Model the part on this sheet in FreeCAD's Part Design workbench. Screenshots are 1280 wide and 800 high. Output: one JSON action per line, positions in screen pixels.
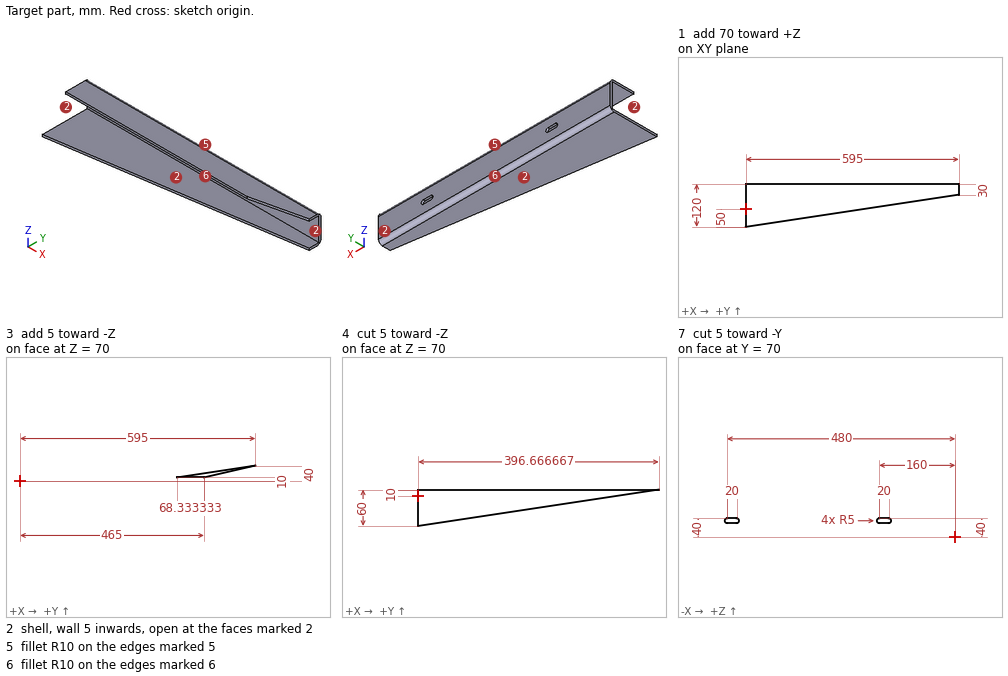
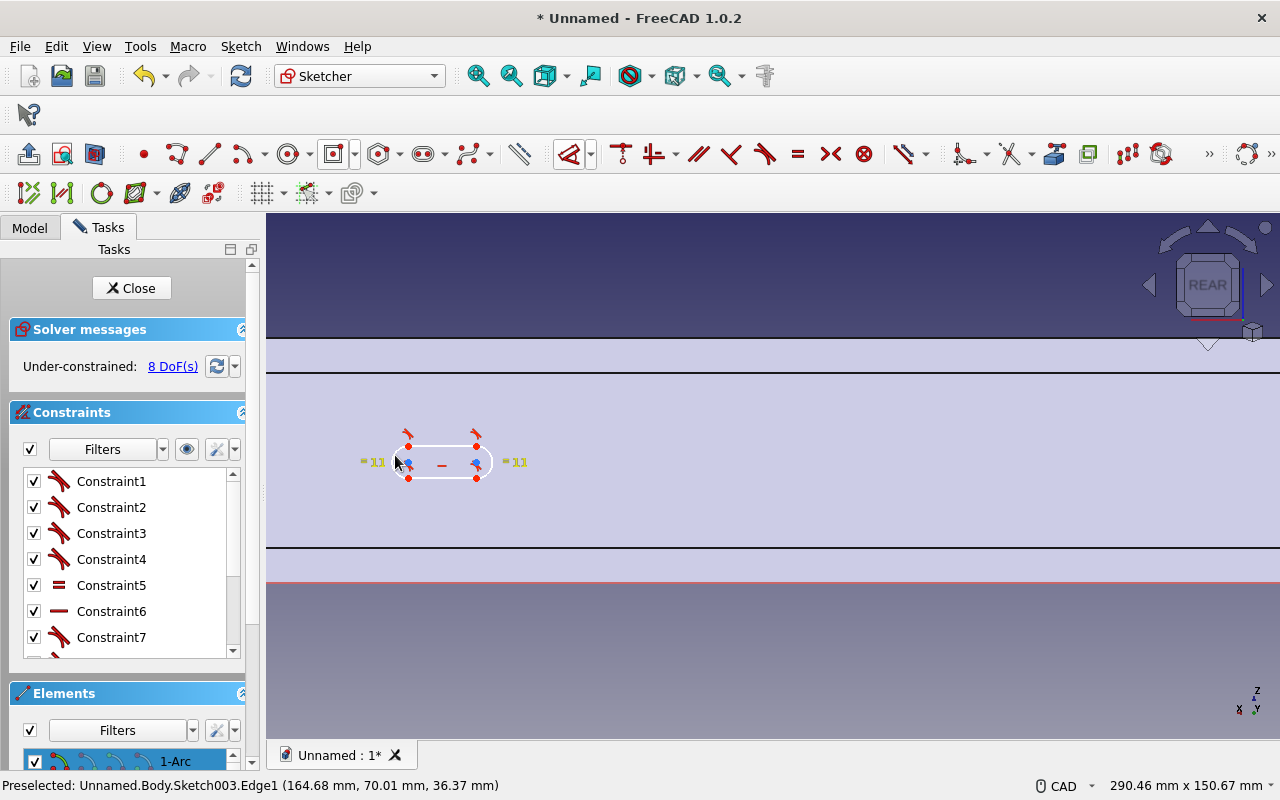
{"action": "left_click", "coordinate": [395, 453]}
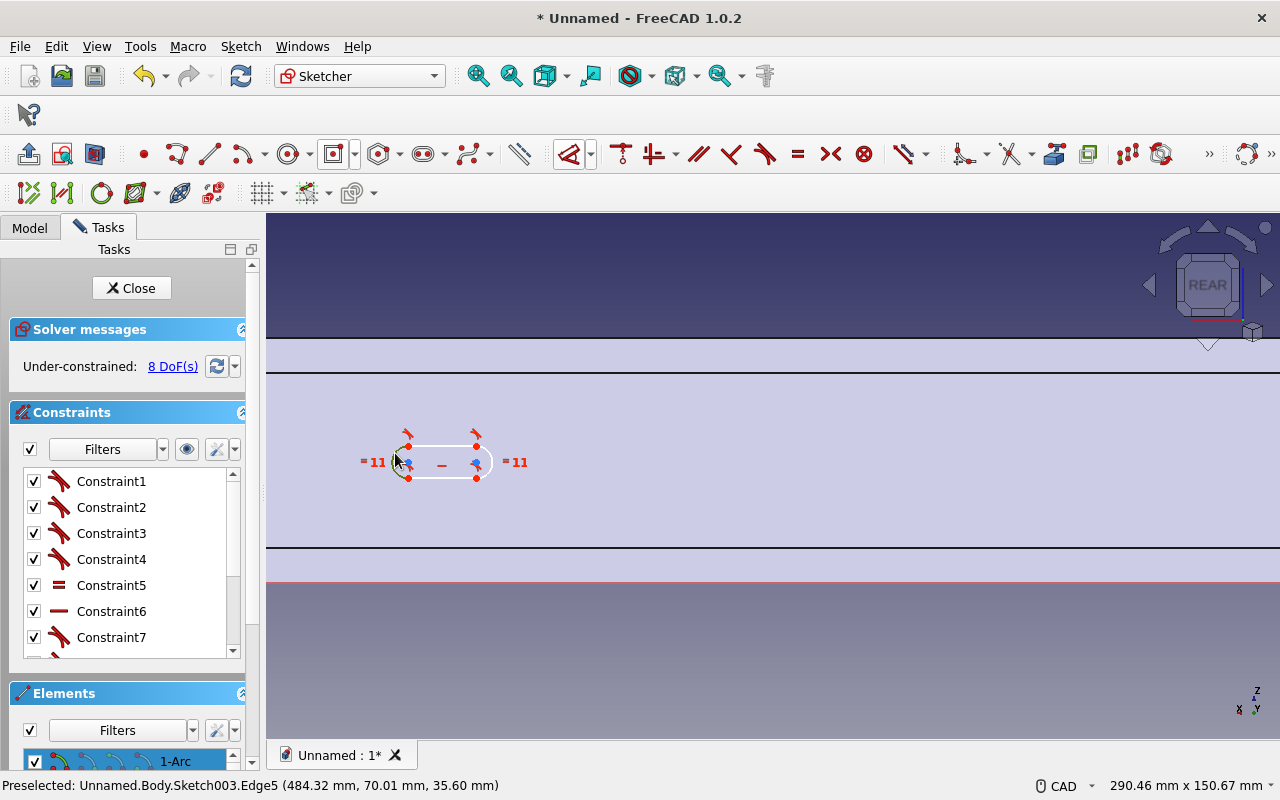
{"action": "left_click", "coordinate": [798, 154]}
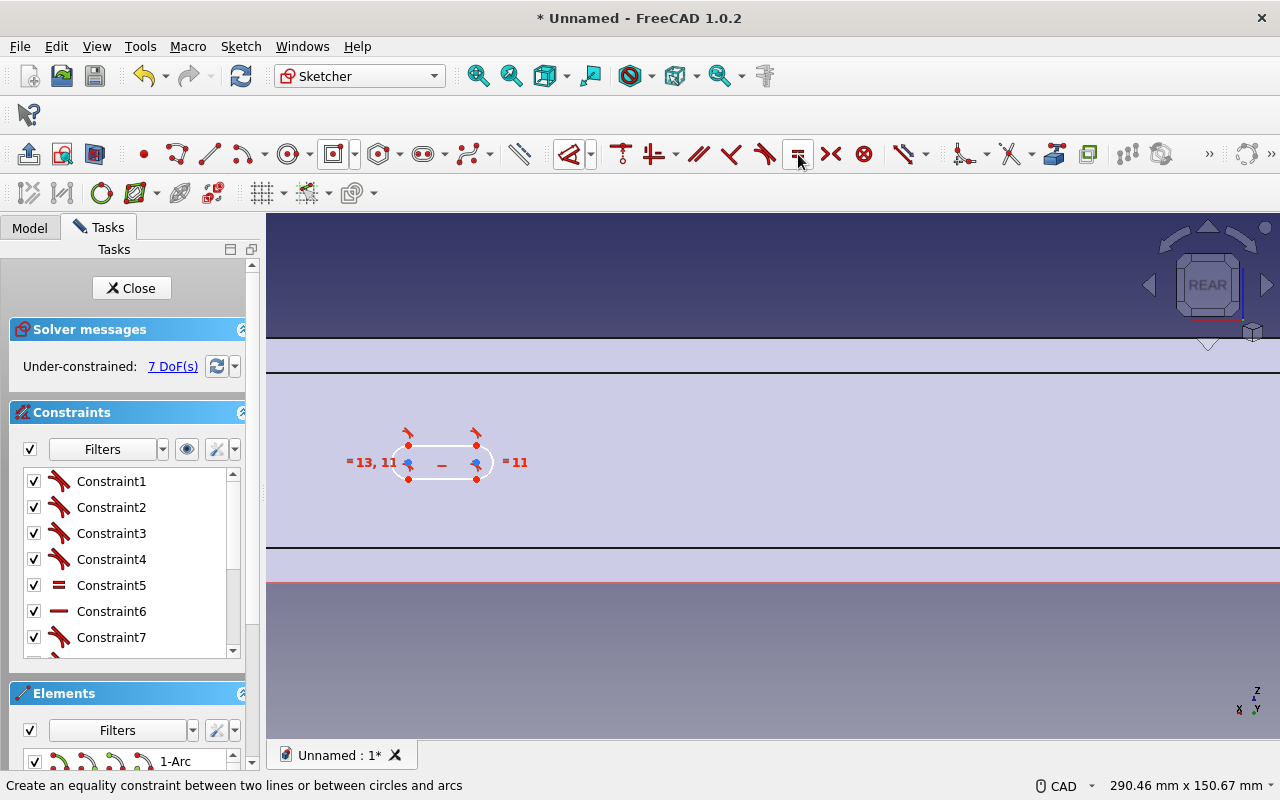
{"action": "scroll", "coordinate": [395, 455], "scroll_direction": "down", "scroll_amount": 5}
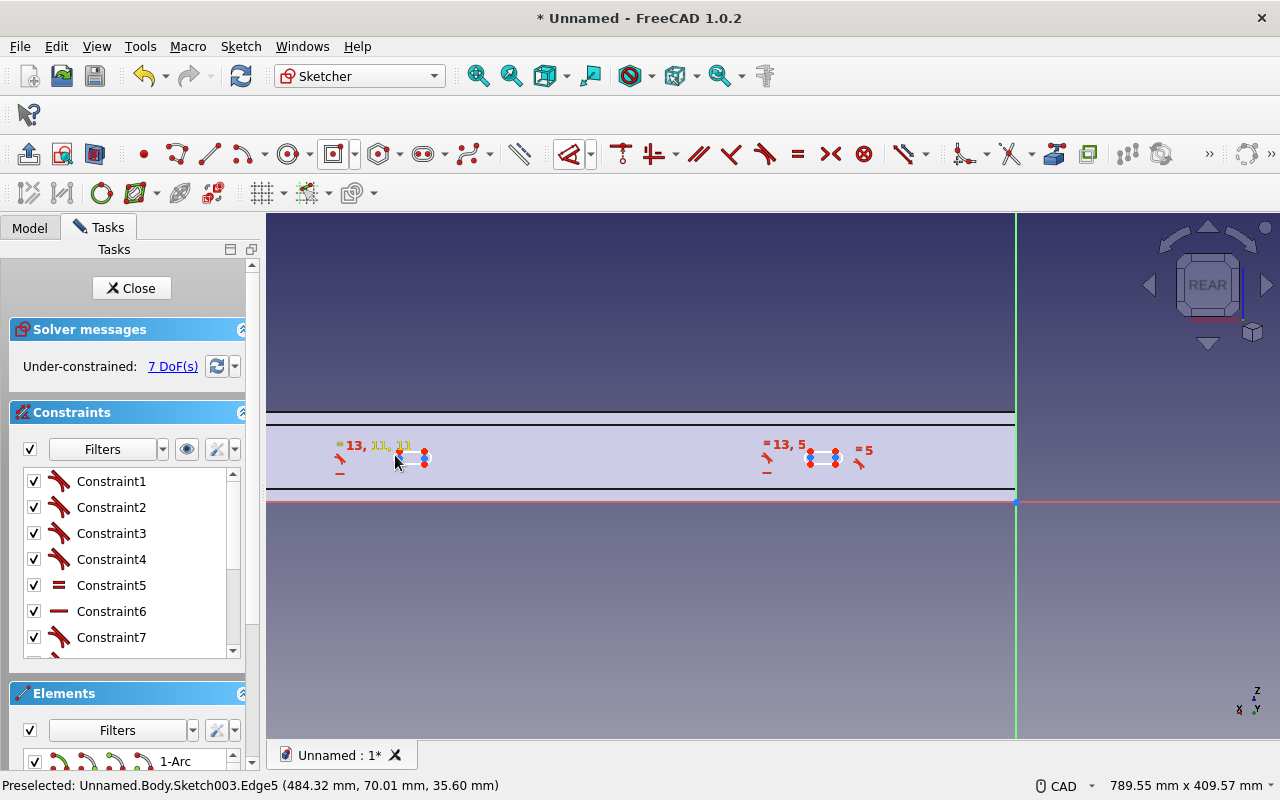
{"action": "scroll", "coordinate": [806, 454], "scroll_direction": "up", "scroll_amount": 10}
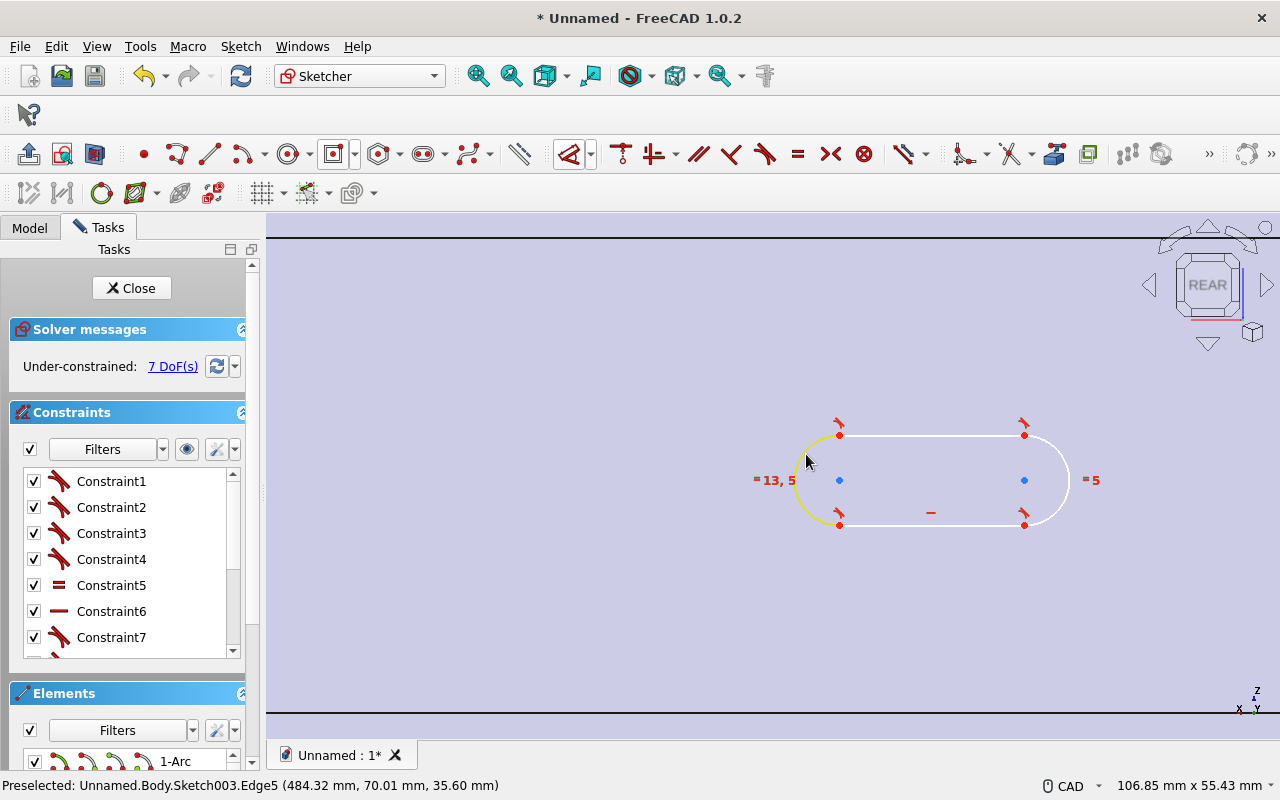
{"action": "left_click", "coordinate": [803, 454]}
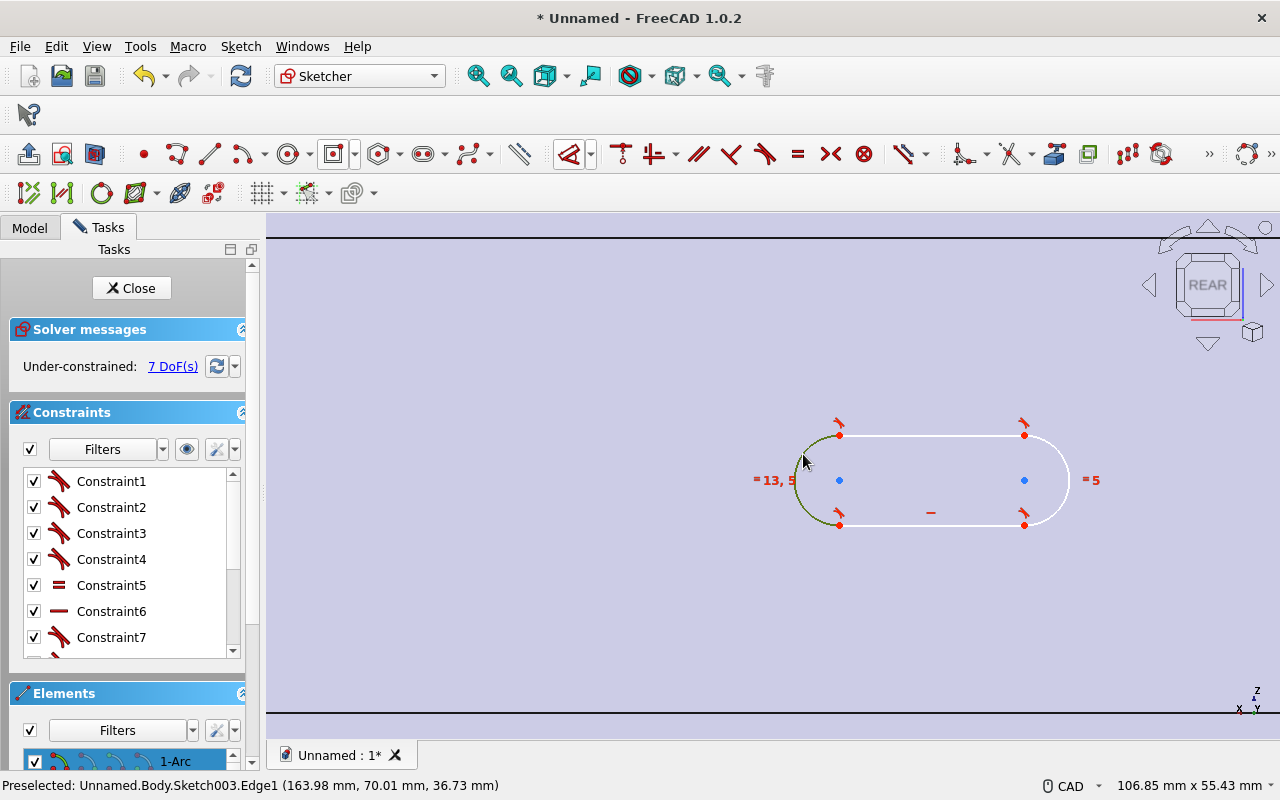
{"action": "left_click", "coordinate": [590, 154]}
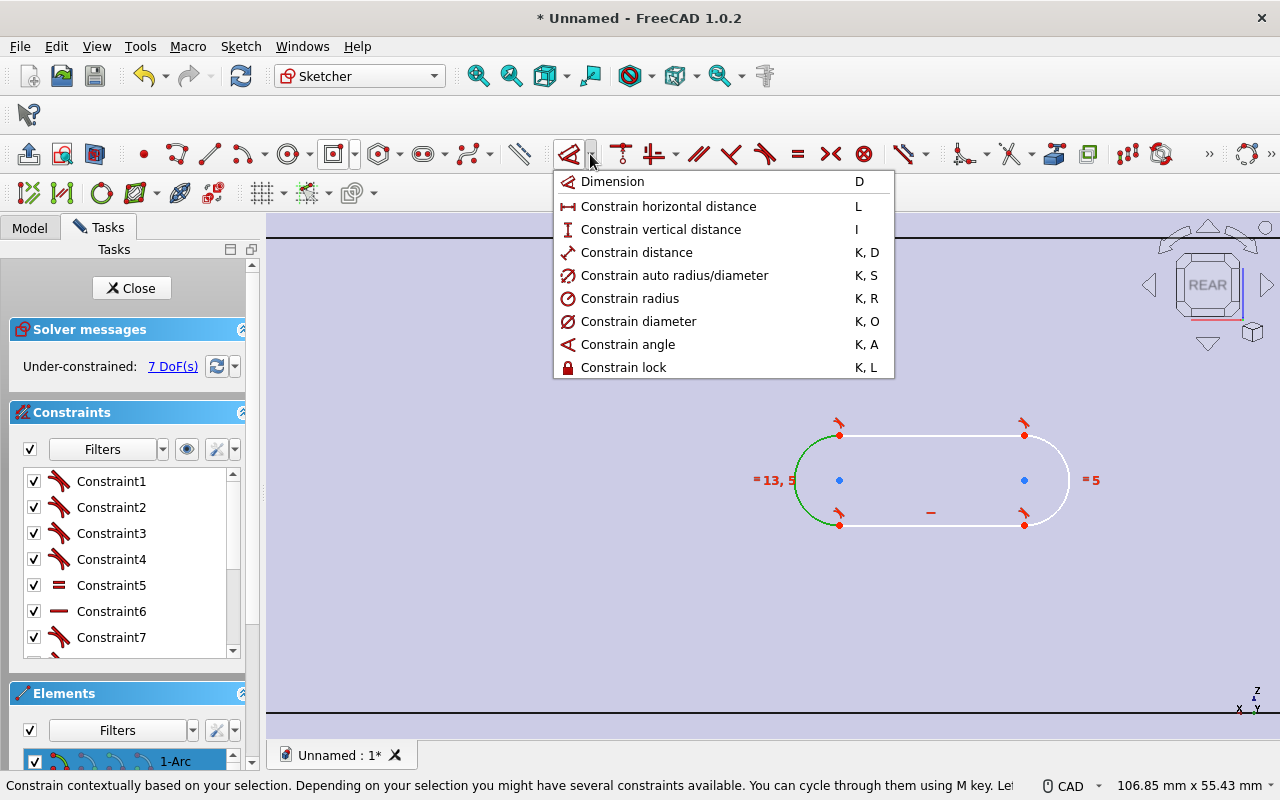
{"action": "left_click", "coordinate": [724, 298]}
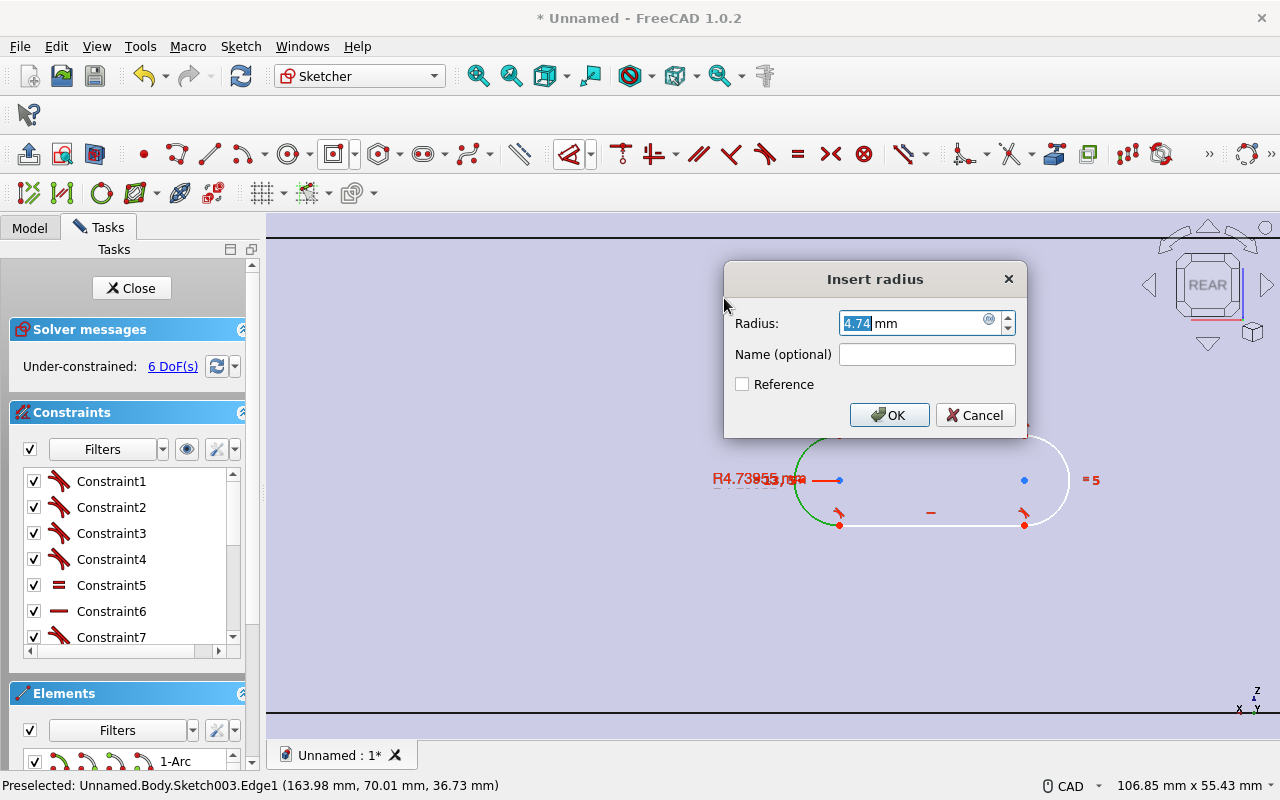
{"action": "type", "text": "5"}
{"action": "key", "text": "Return"}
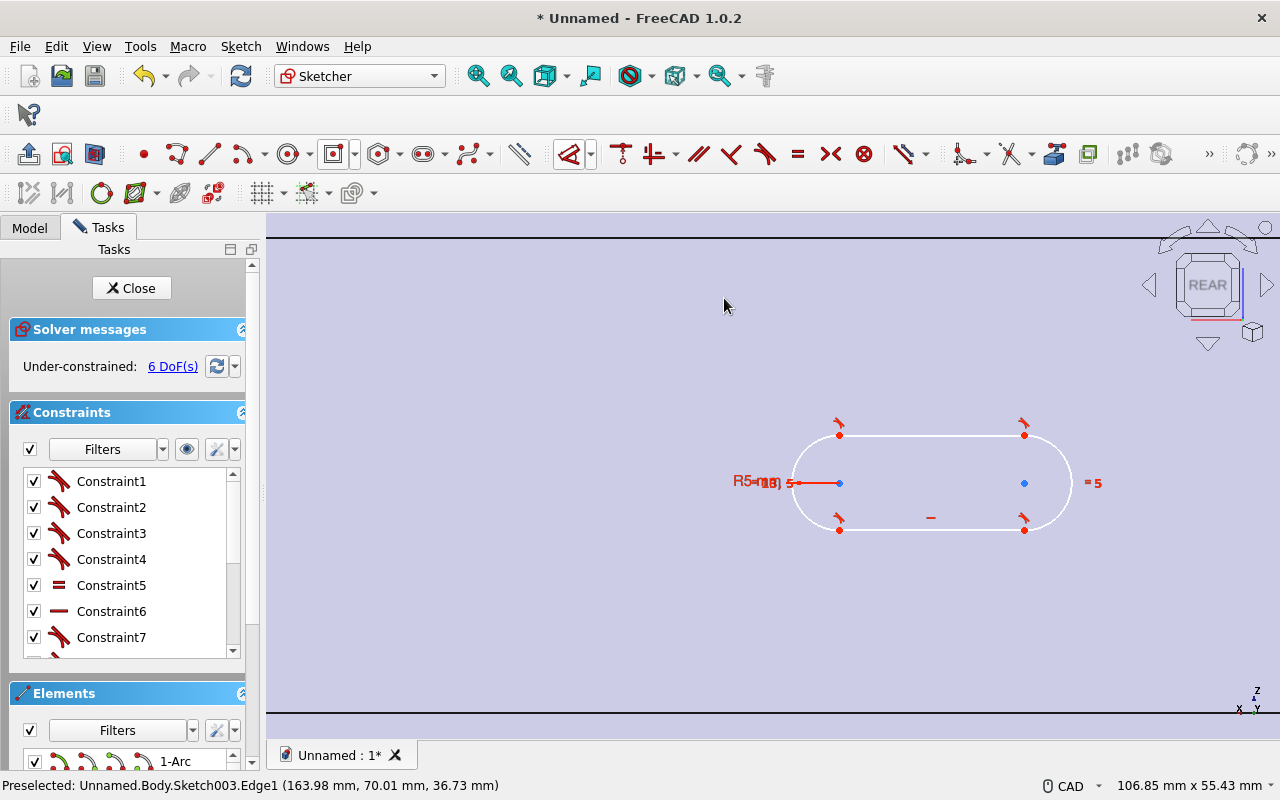
{"action": "scroll", "coordinate": [806, 454], "scroll_direction": "down", "scroll_amount": 10}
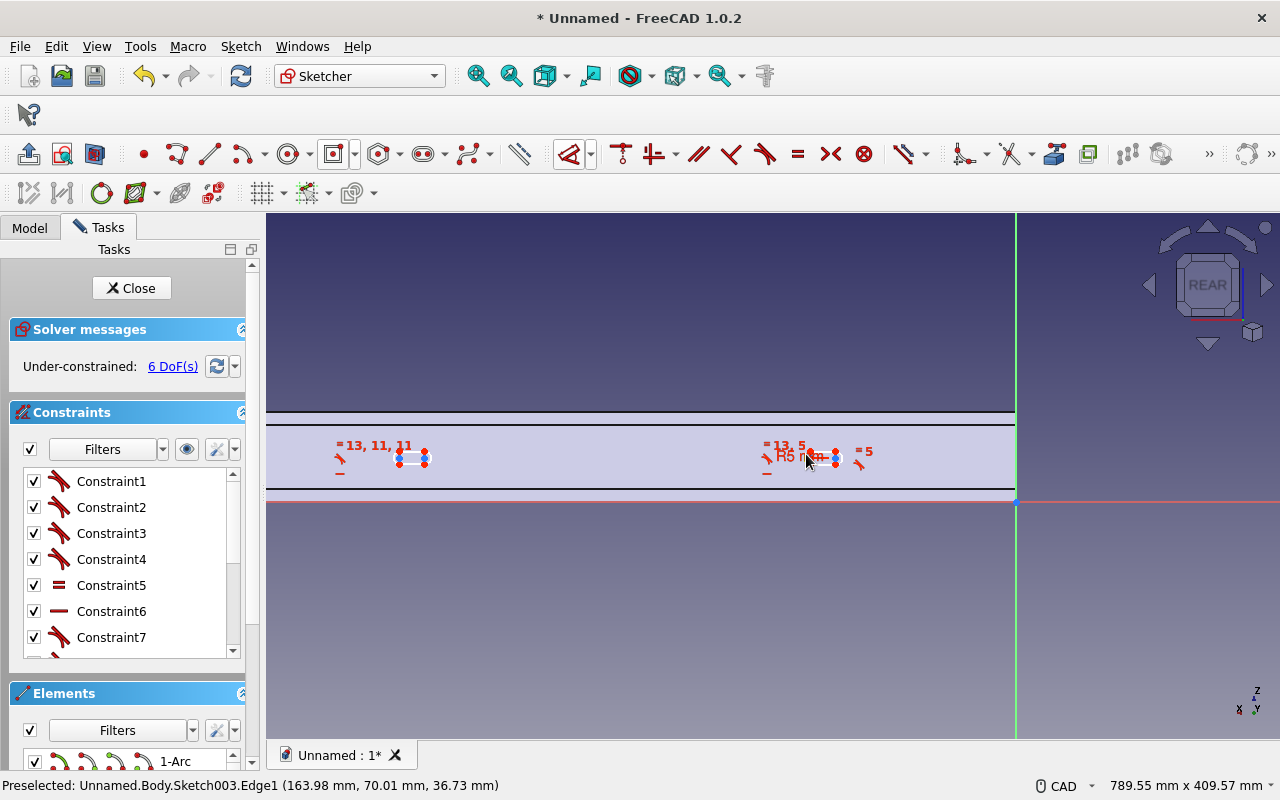
{"action": "scroll", "coordinate": [818, 452], "scroll_direction": "up", "scroll_amount": 4}